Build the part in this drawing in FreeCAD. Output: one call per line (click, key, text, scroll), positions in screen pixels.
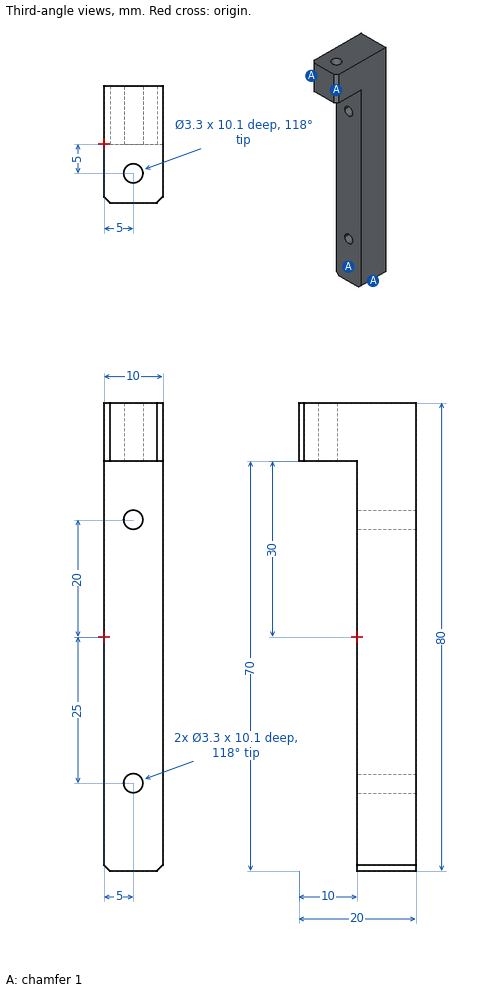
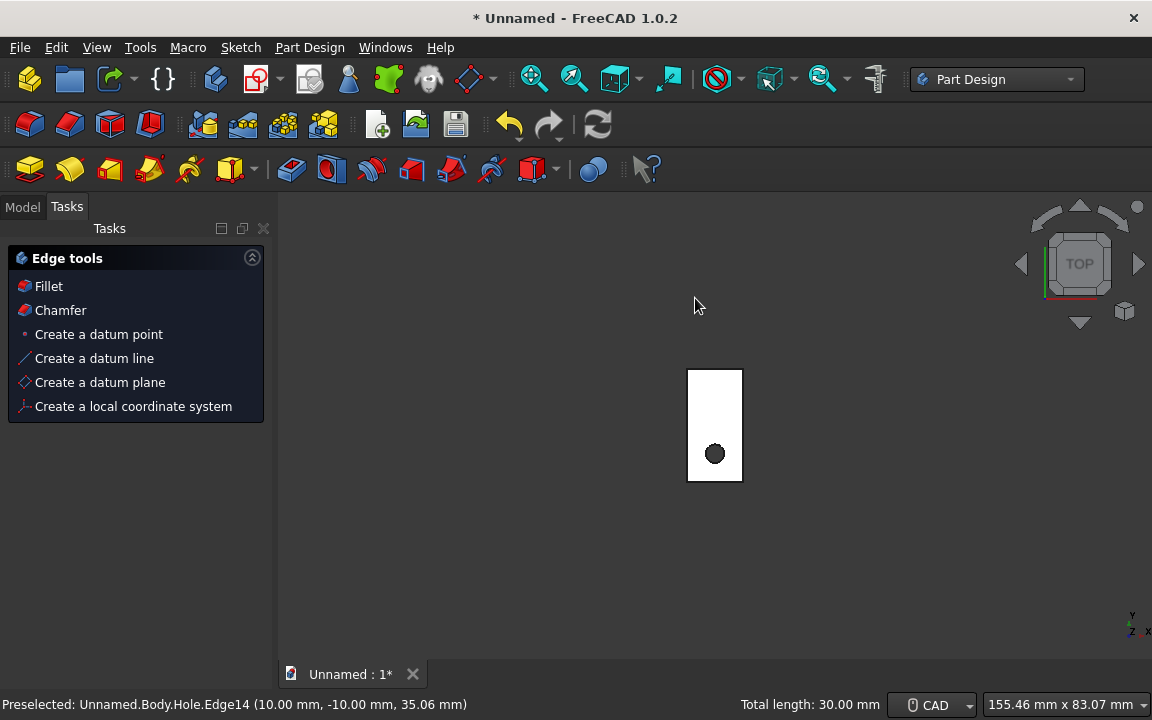
key(1)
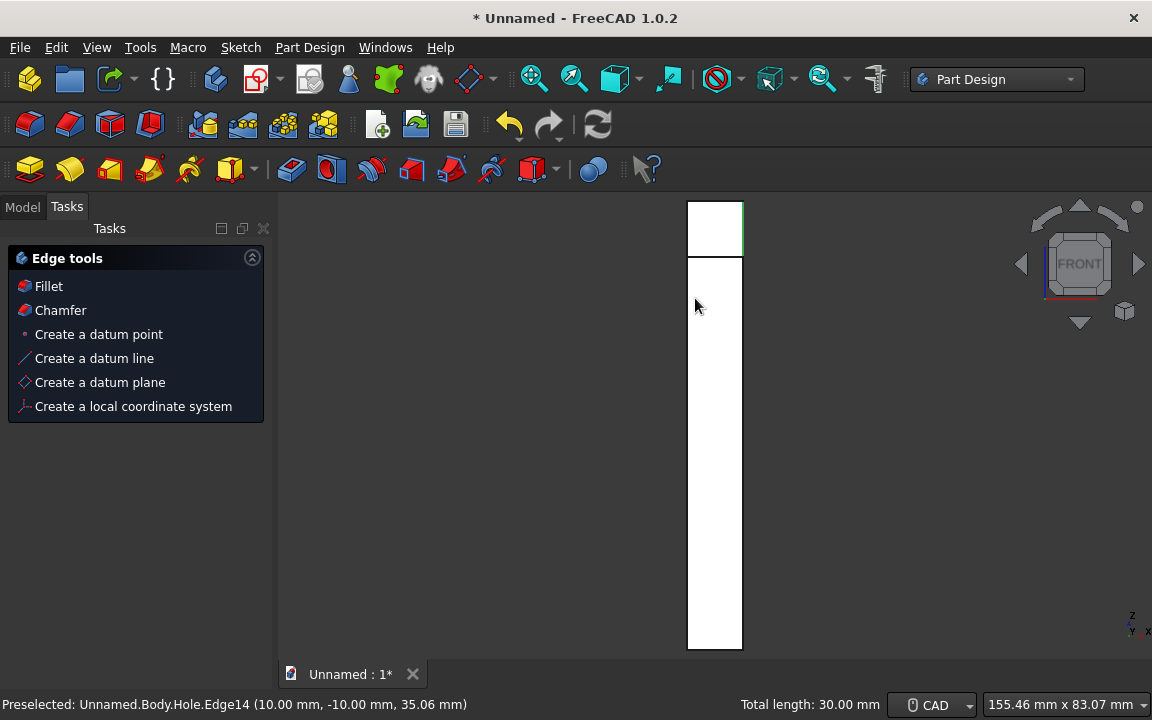
click(687, 228, ctrl)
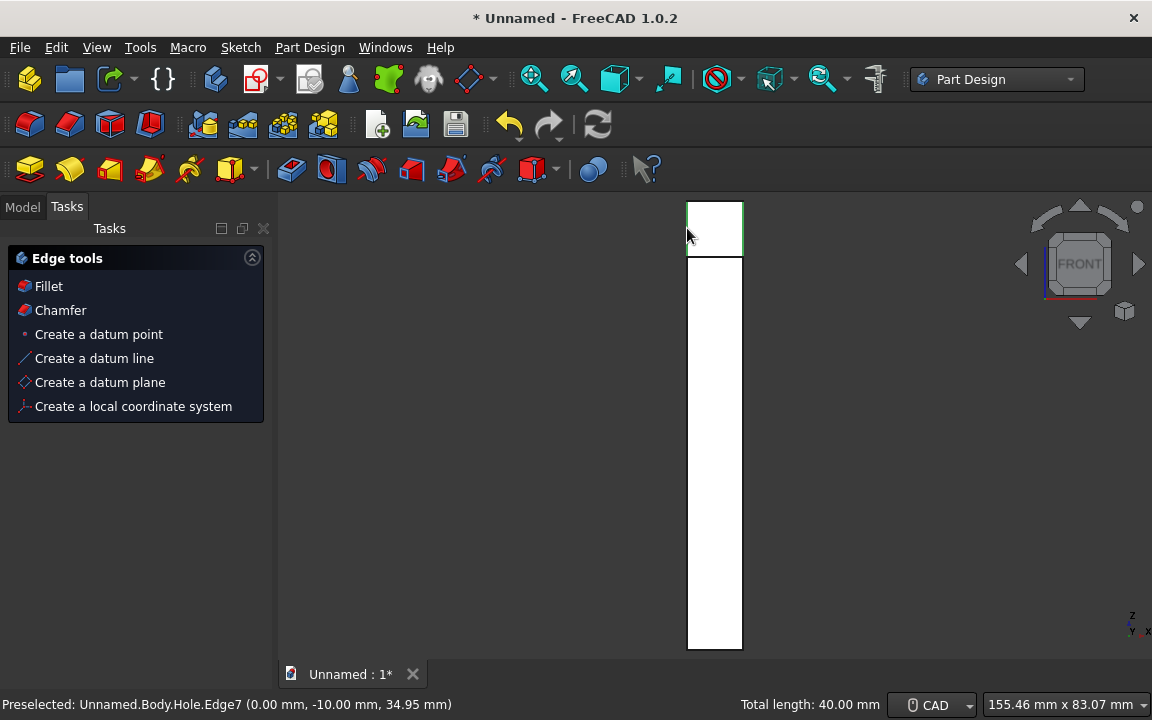
click(70, 124)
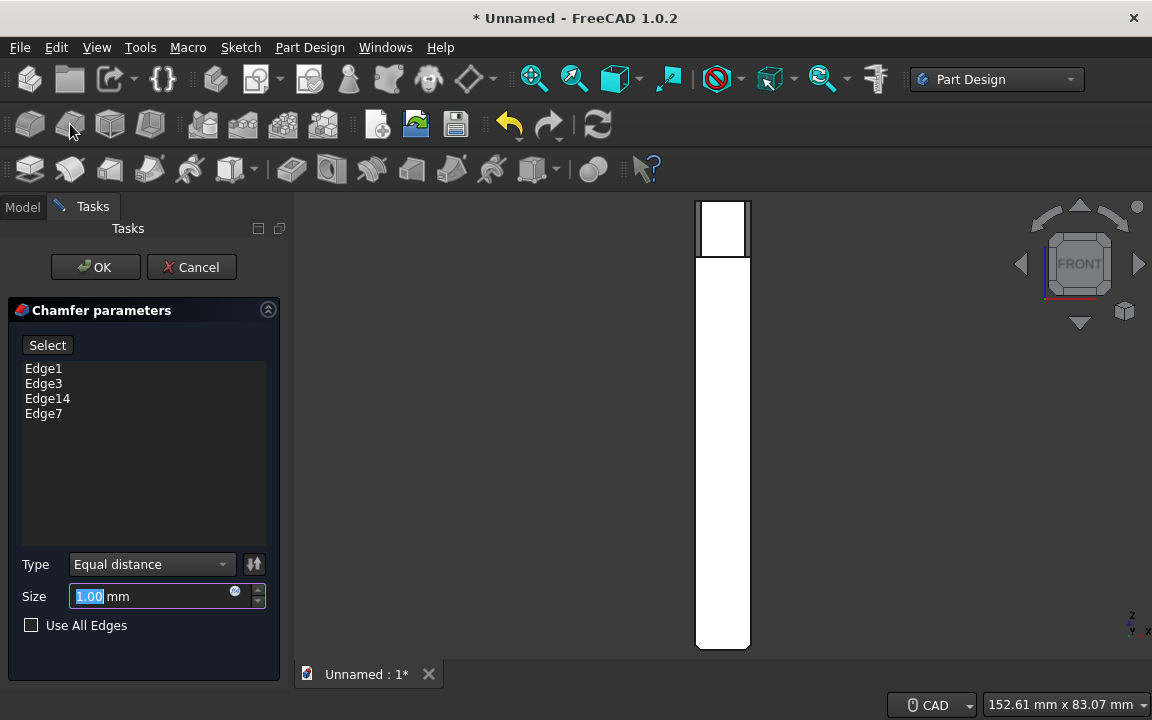
text(1)
key(Tab)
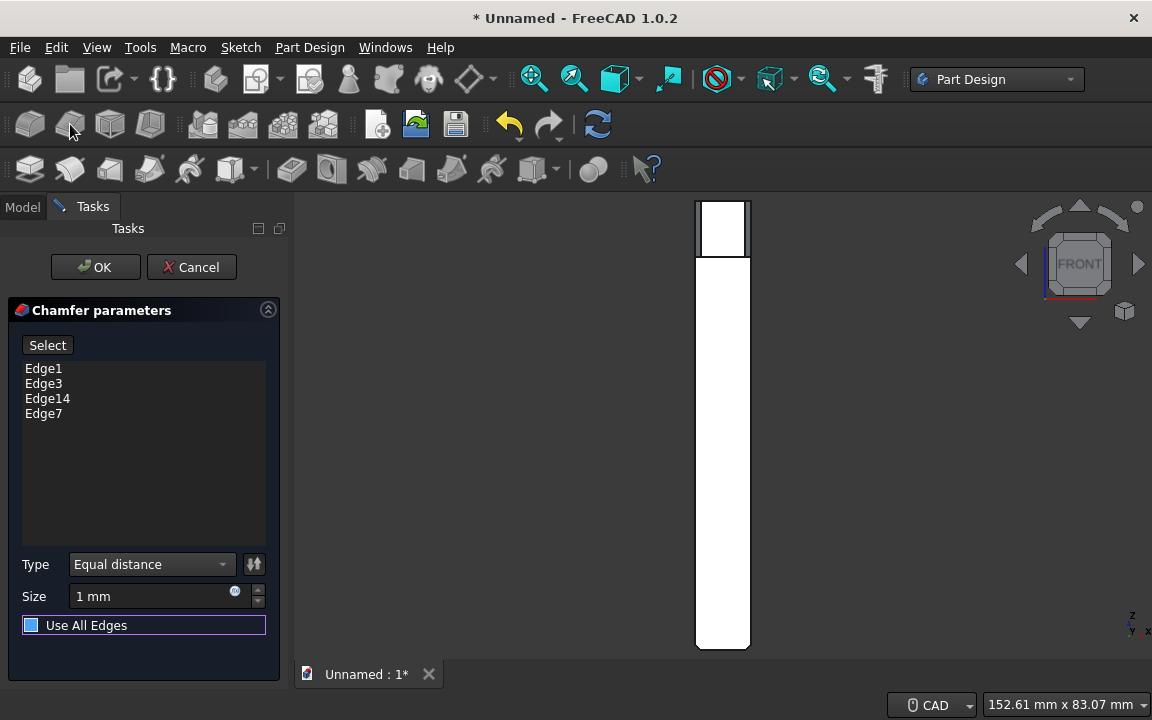
click(96, 267)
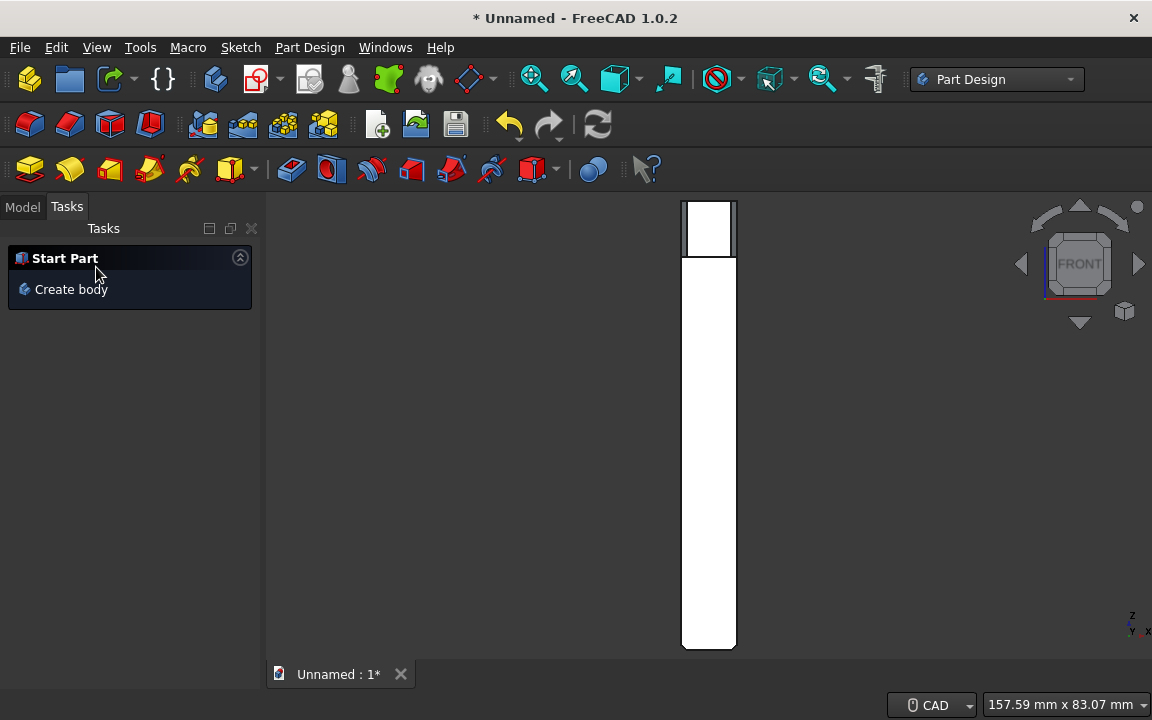
key(4)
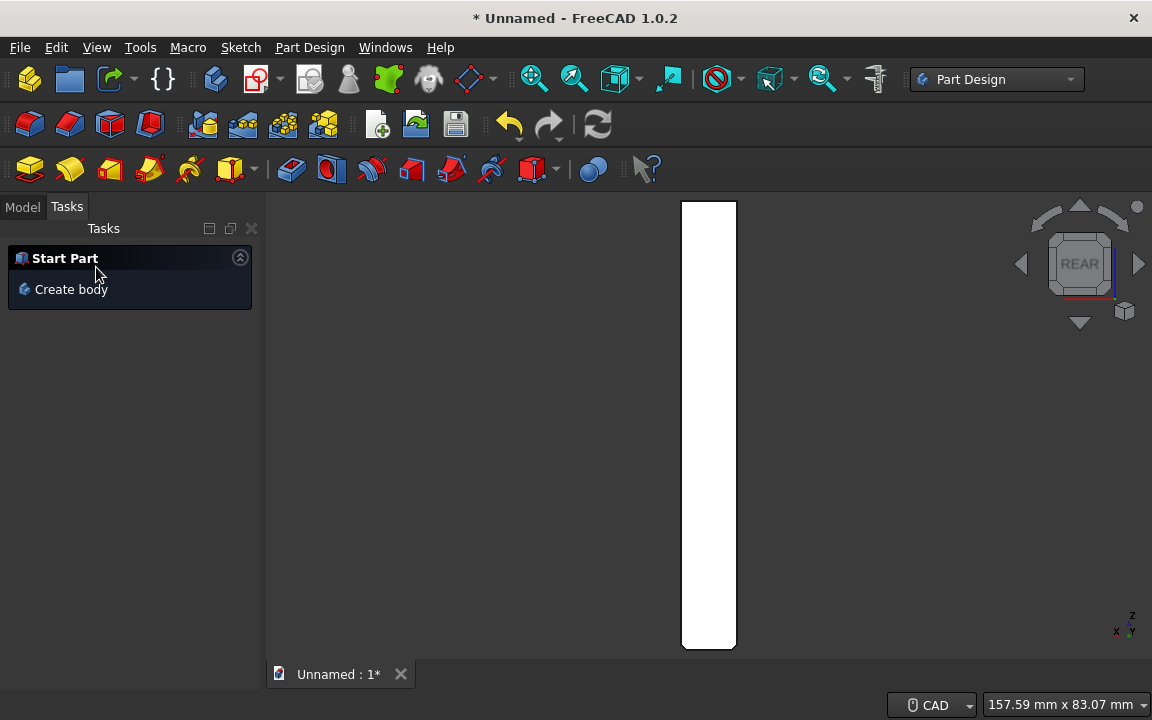
click(709, 617)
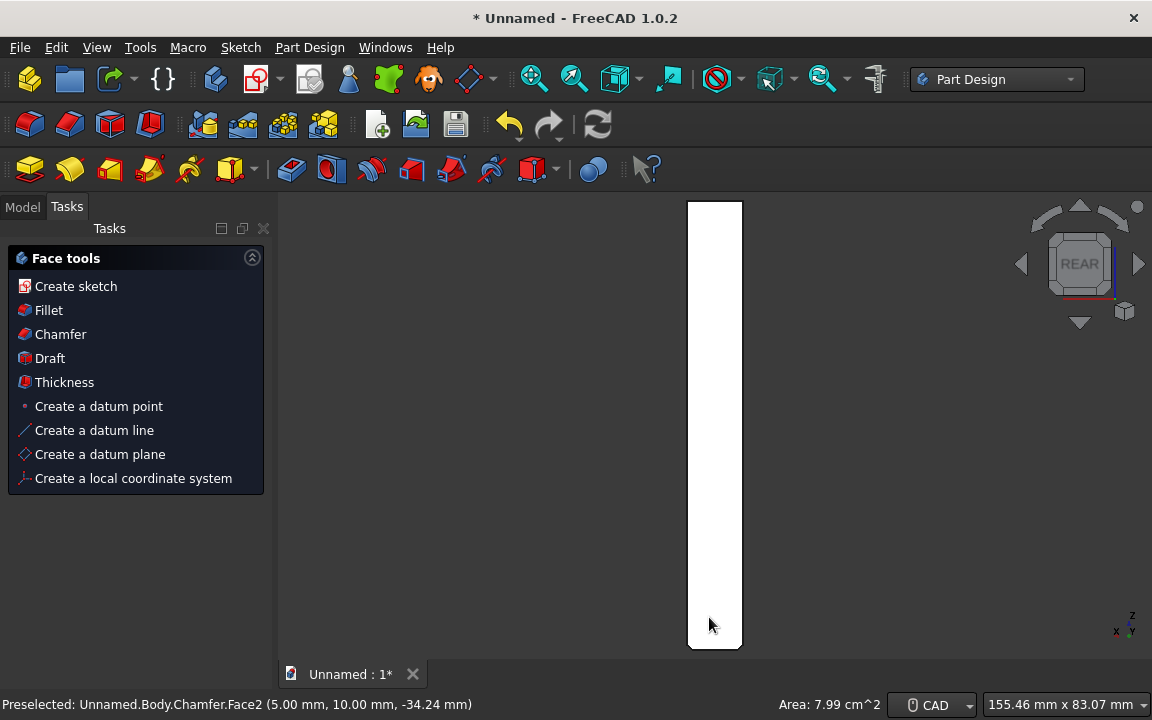
click(256, 80)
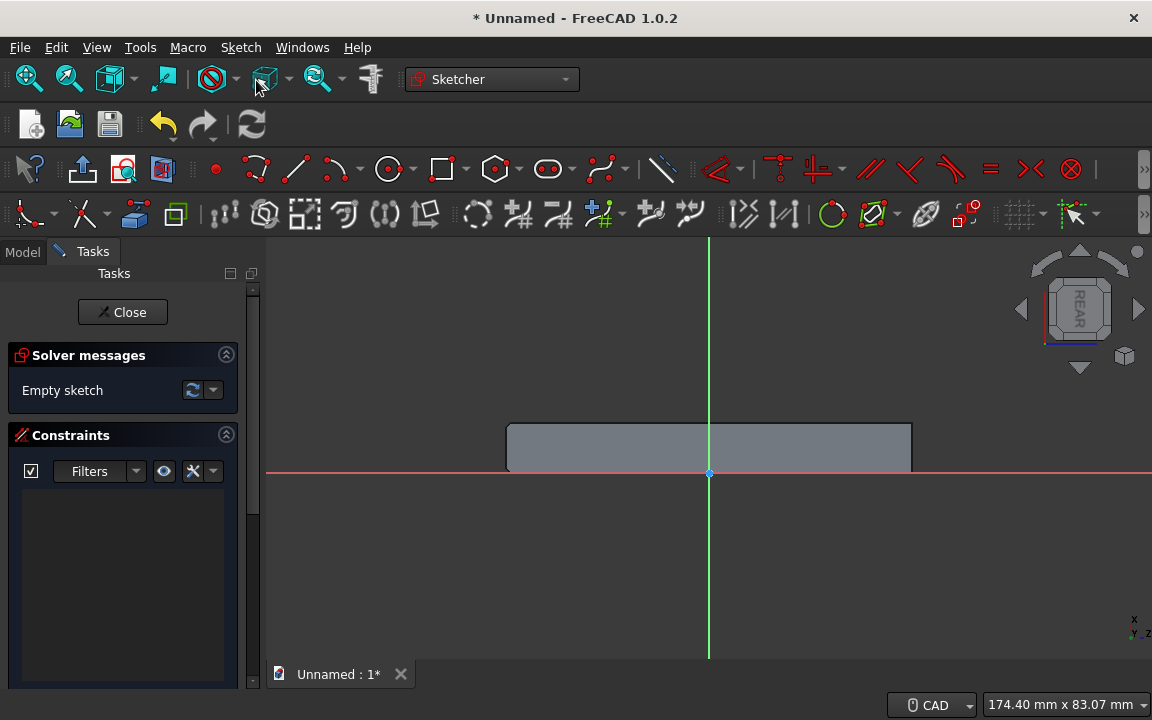
scroll(764, 467, up, 3)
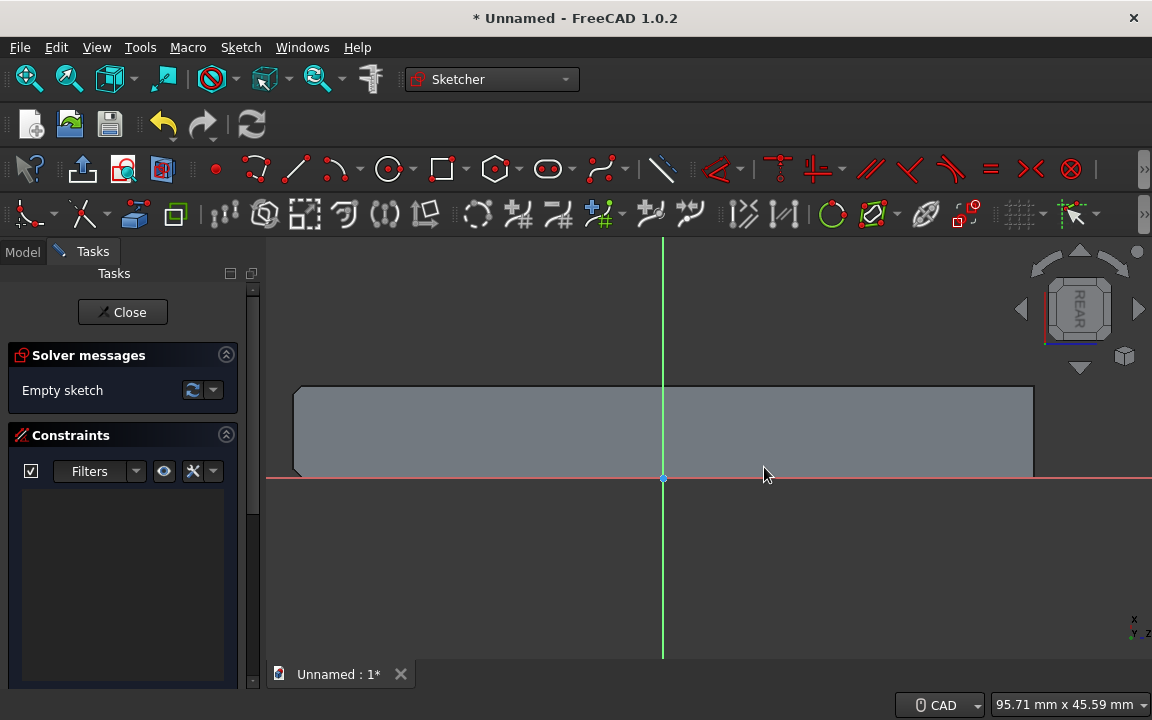
key(g)
key(c)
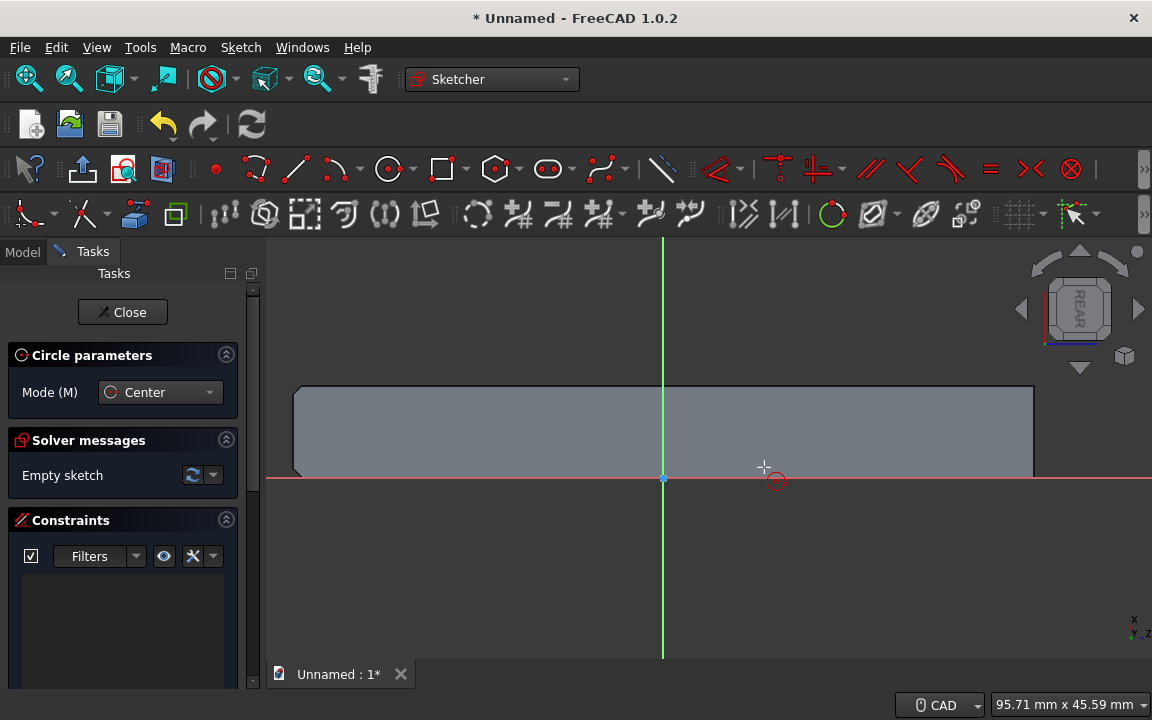
scroll(432, 432, up, 2)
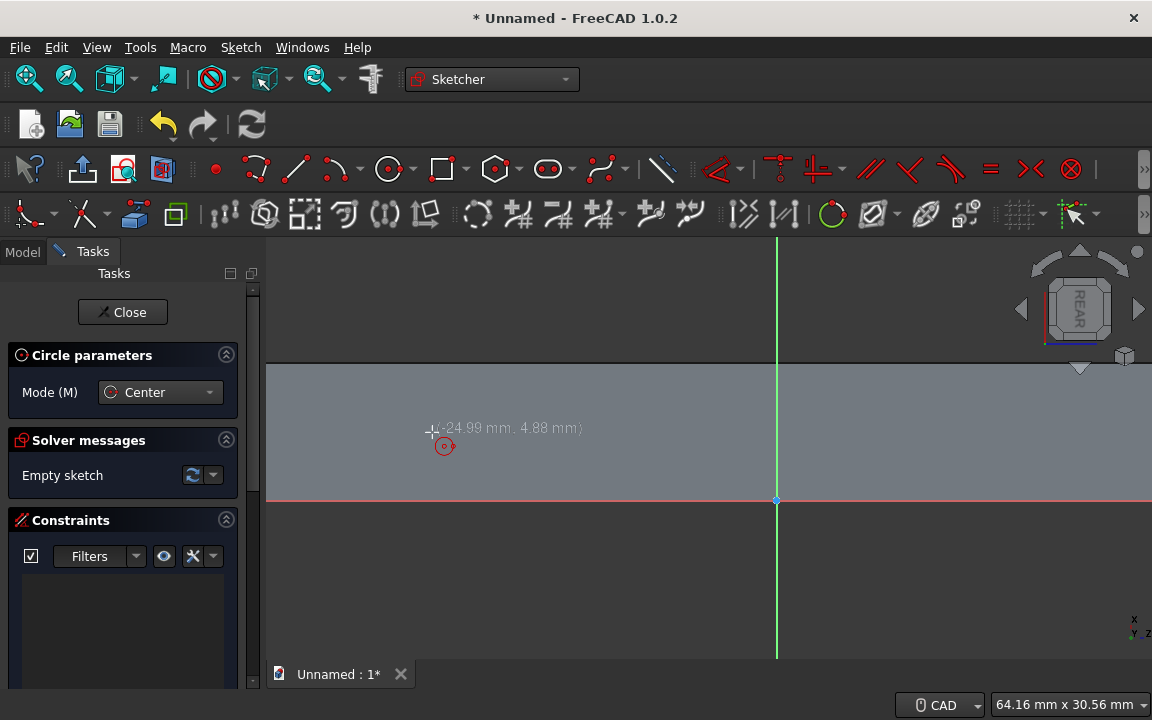
click(432, 432)
move(448, 416)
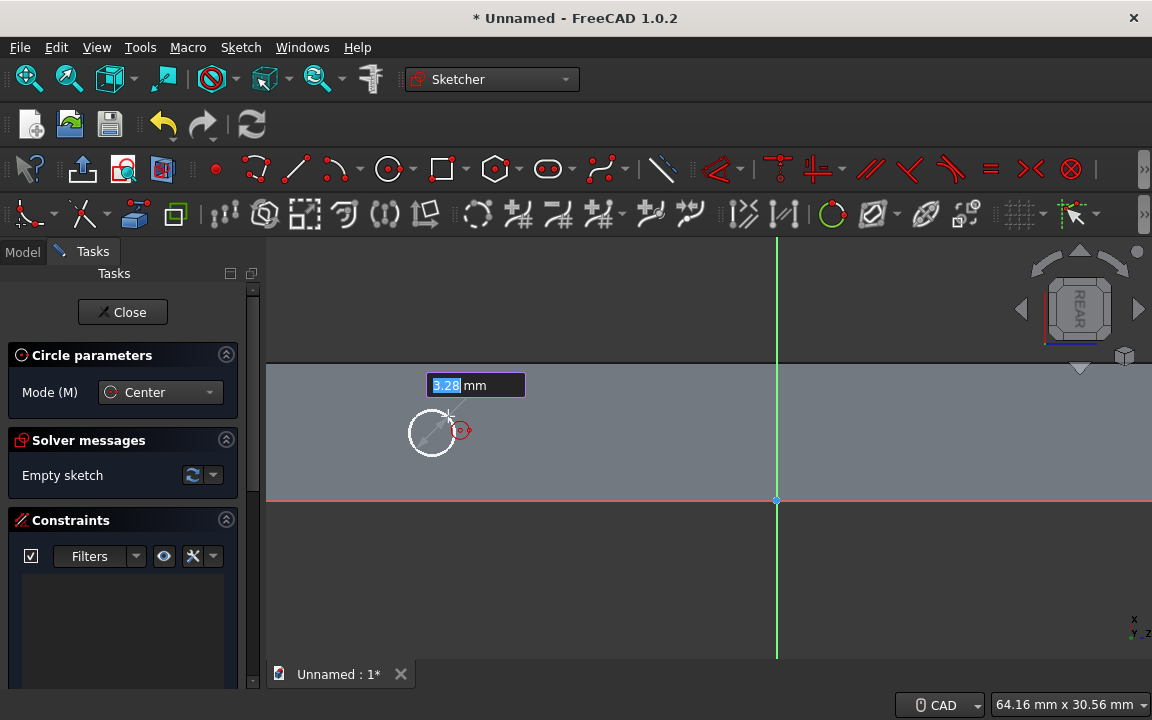
text(3.3)
key(Return)